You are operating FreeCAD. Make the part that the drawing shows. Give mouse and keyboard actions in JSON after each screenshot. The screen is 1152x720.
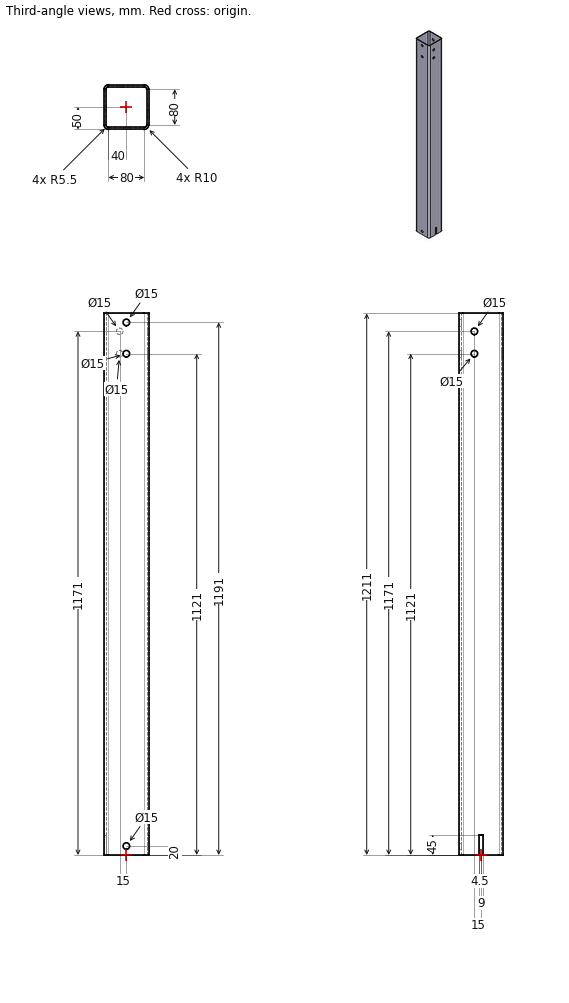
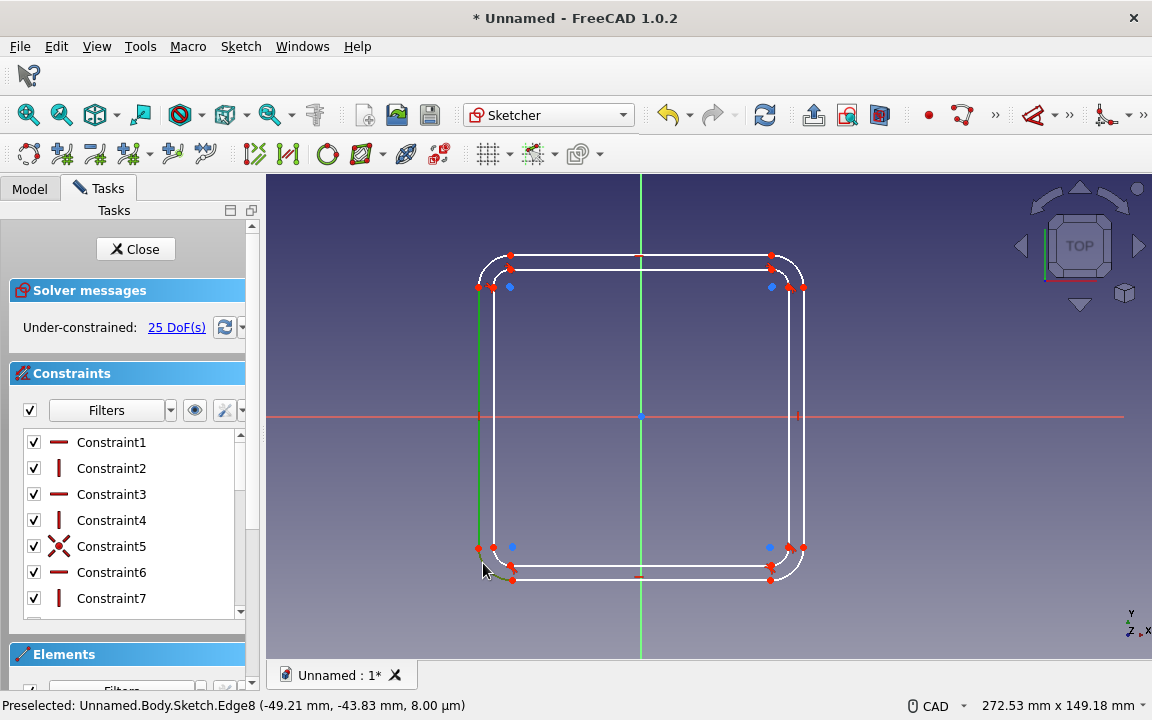
{"action": "key", "text": "t"}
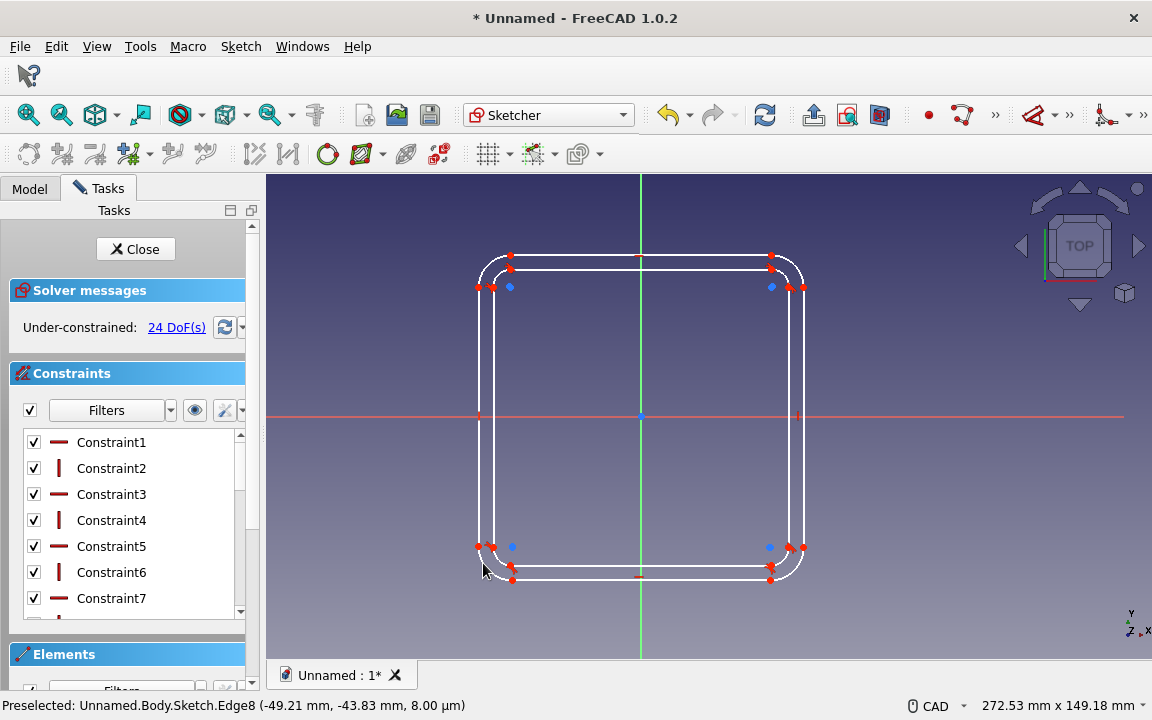
{"action": "left_click", "coordinate": [693, 566]}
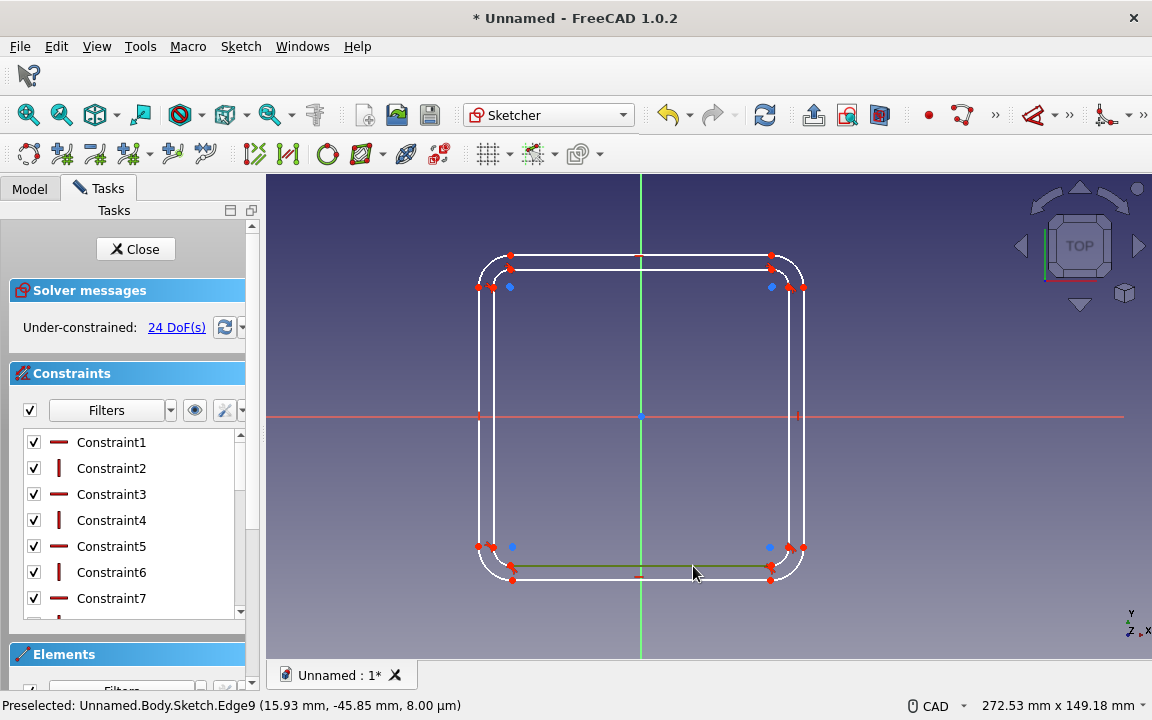
{"action": "left_click", "coordinate": [499, 560]}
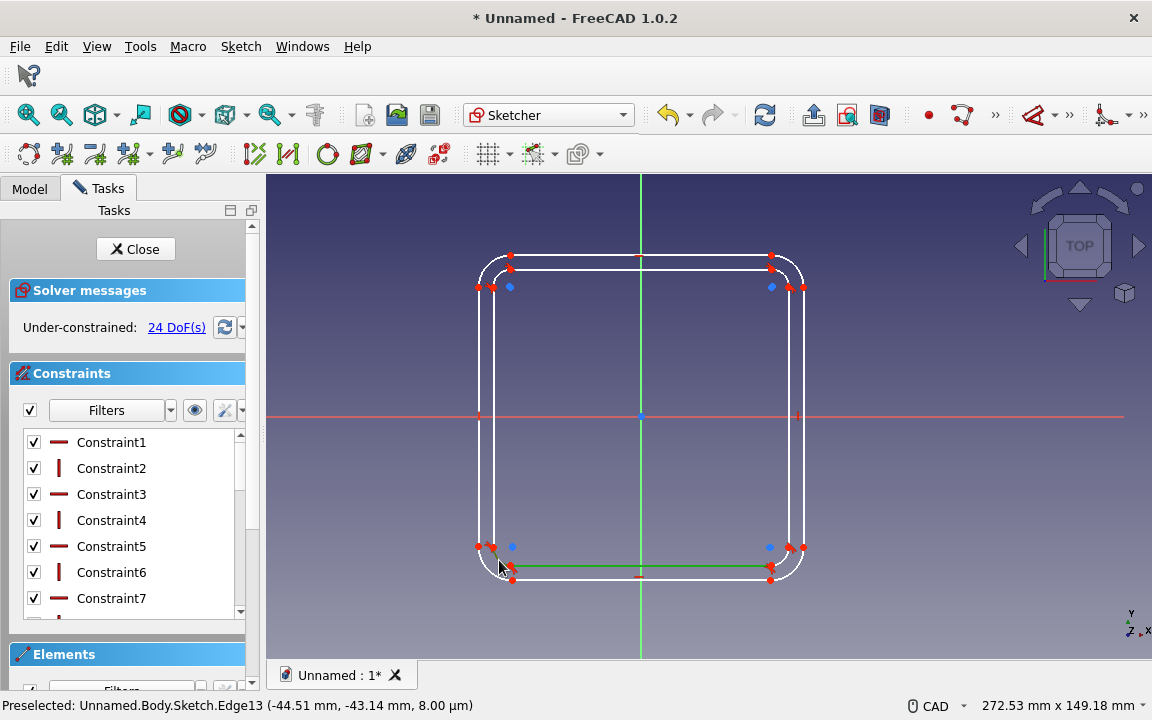
{"action": "key", "text": "t"}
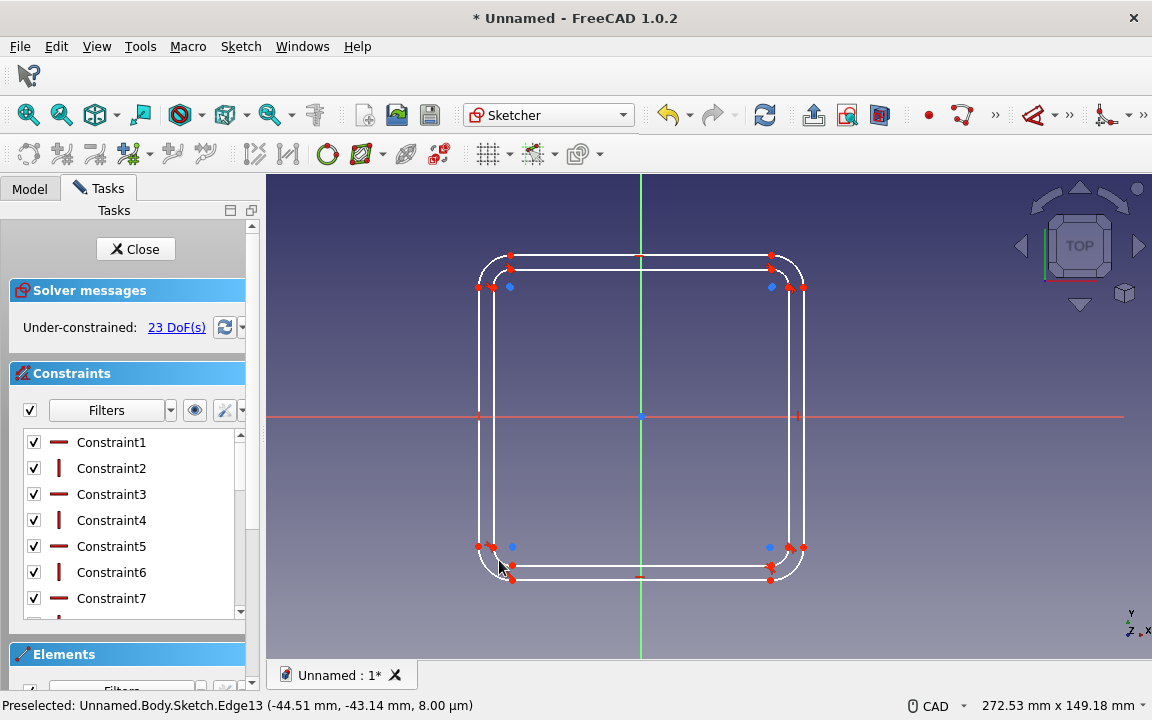
{"action": "left_click", "coordinate": [694, 566]}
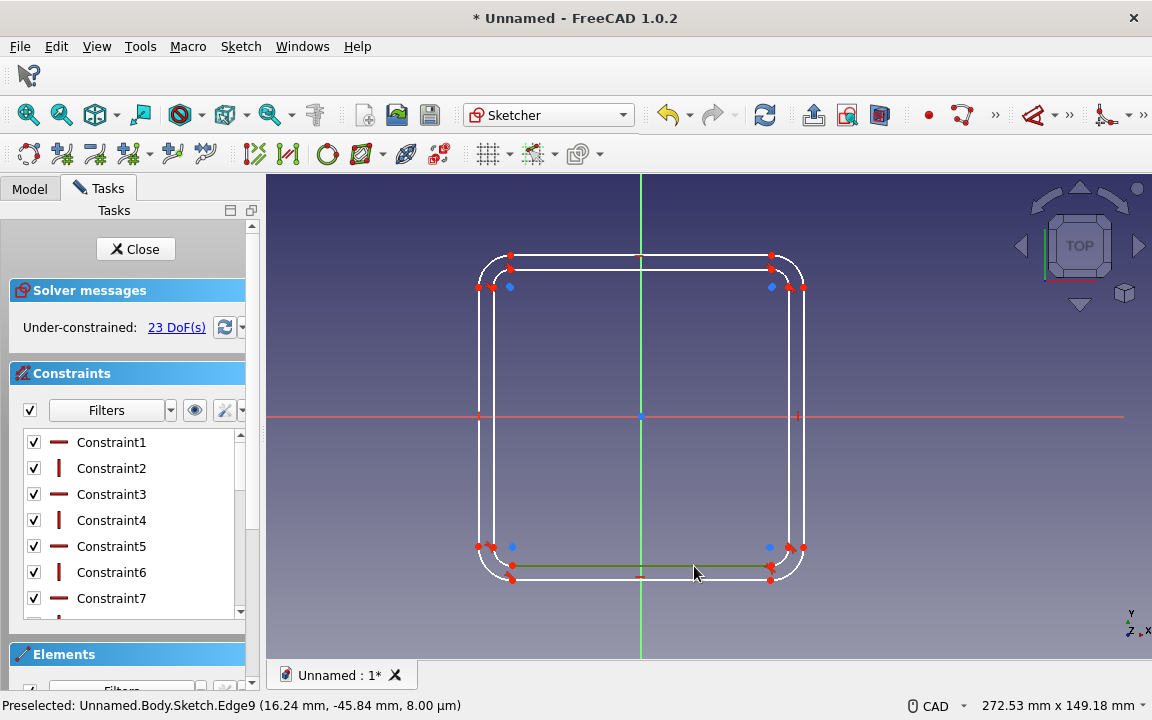
{"action": "left_click", "coordinate": [784, 560]}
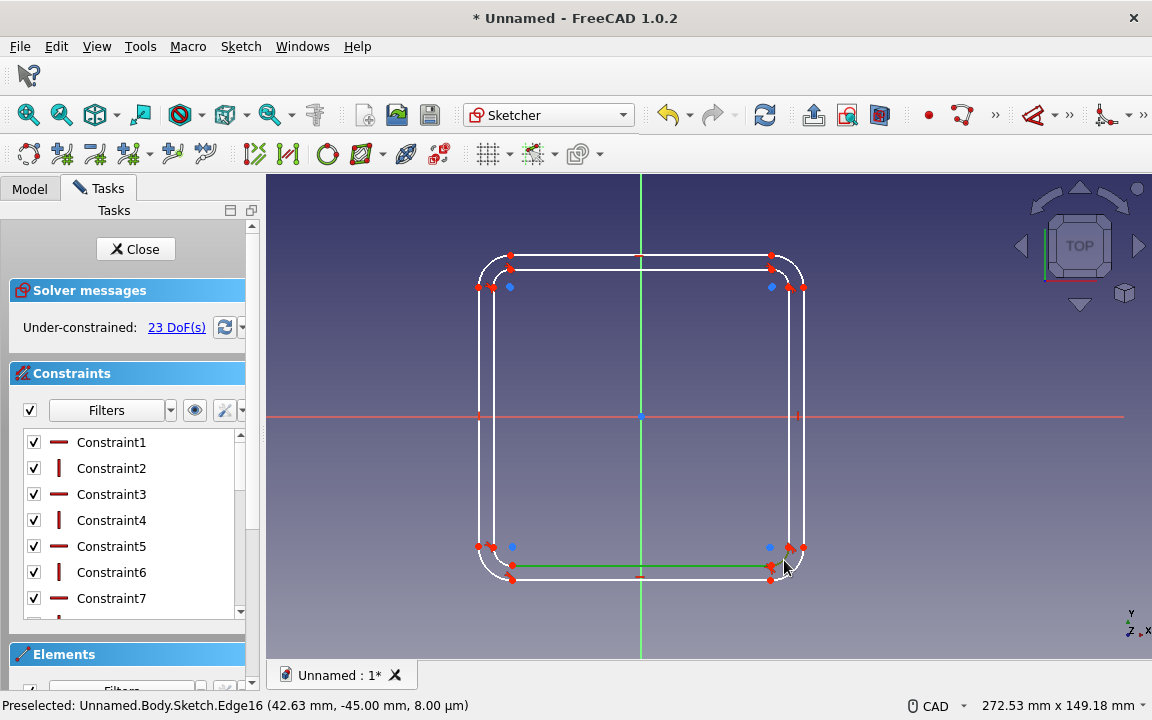
{"action": "key", "text": "t"}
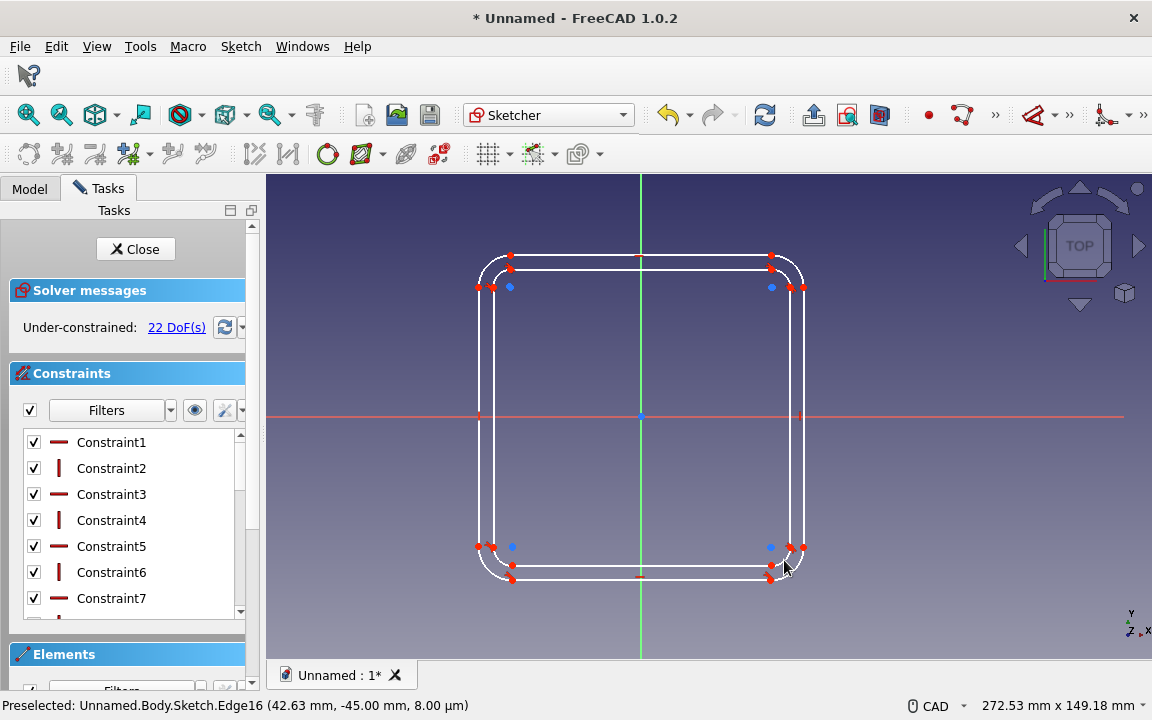
{"action": "left_click", "coordinate": [494, 470]}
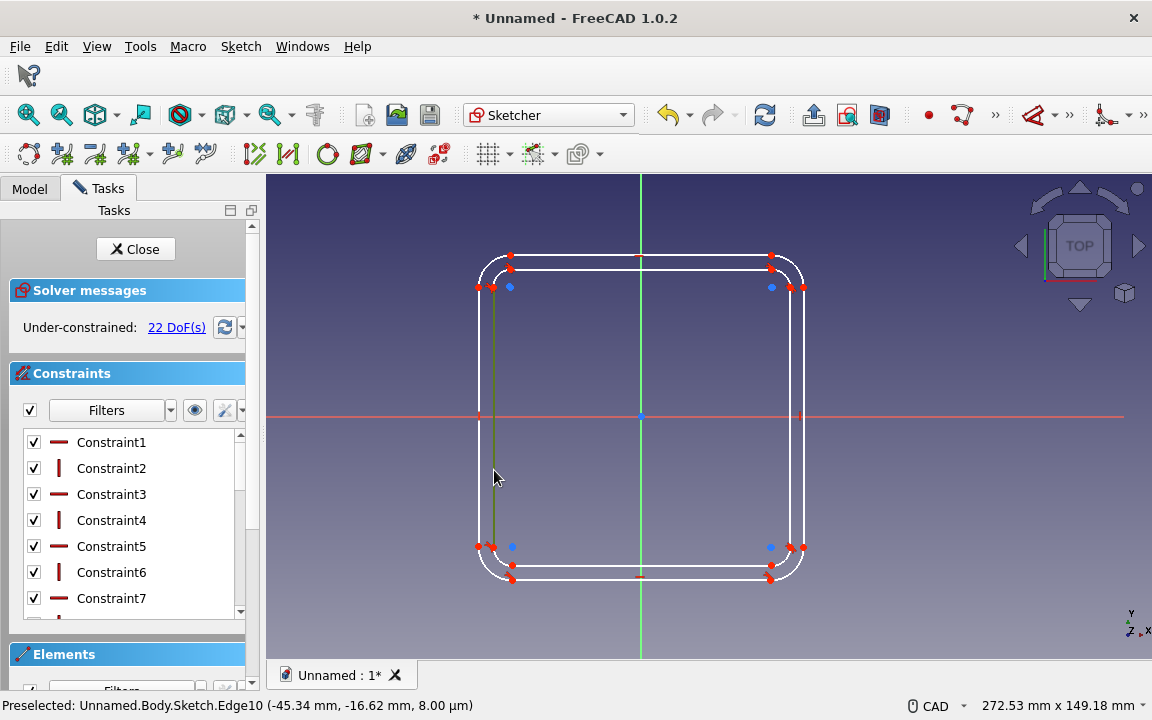
{"action": "left_click", "coordinate": [500, 561]}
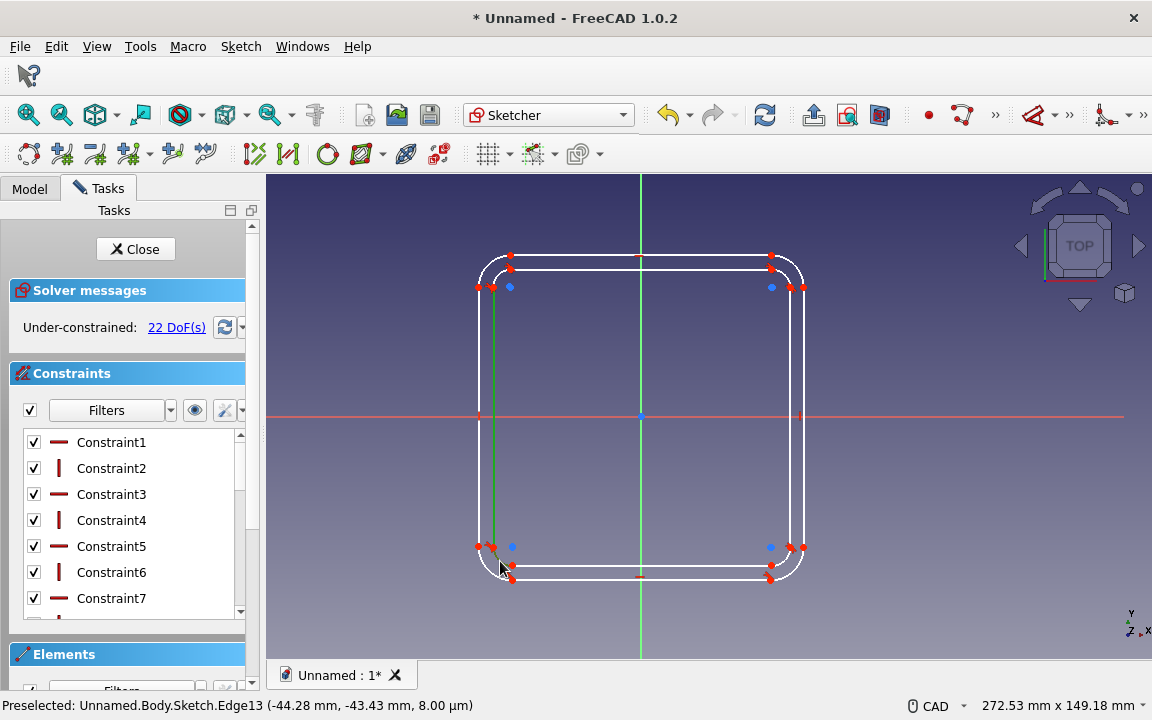
{"action": "key", "text": "t"}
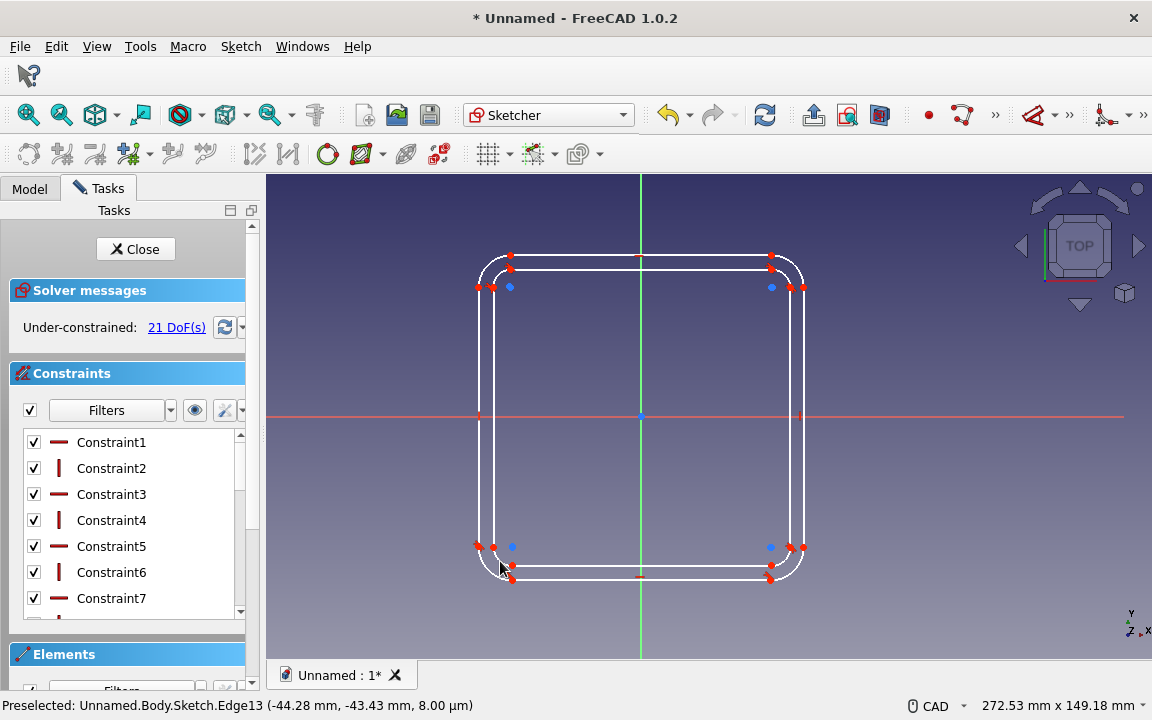
{"action": "left_click", "coordinate": [494, 470]}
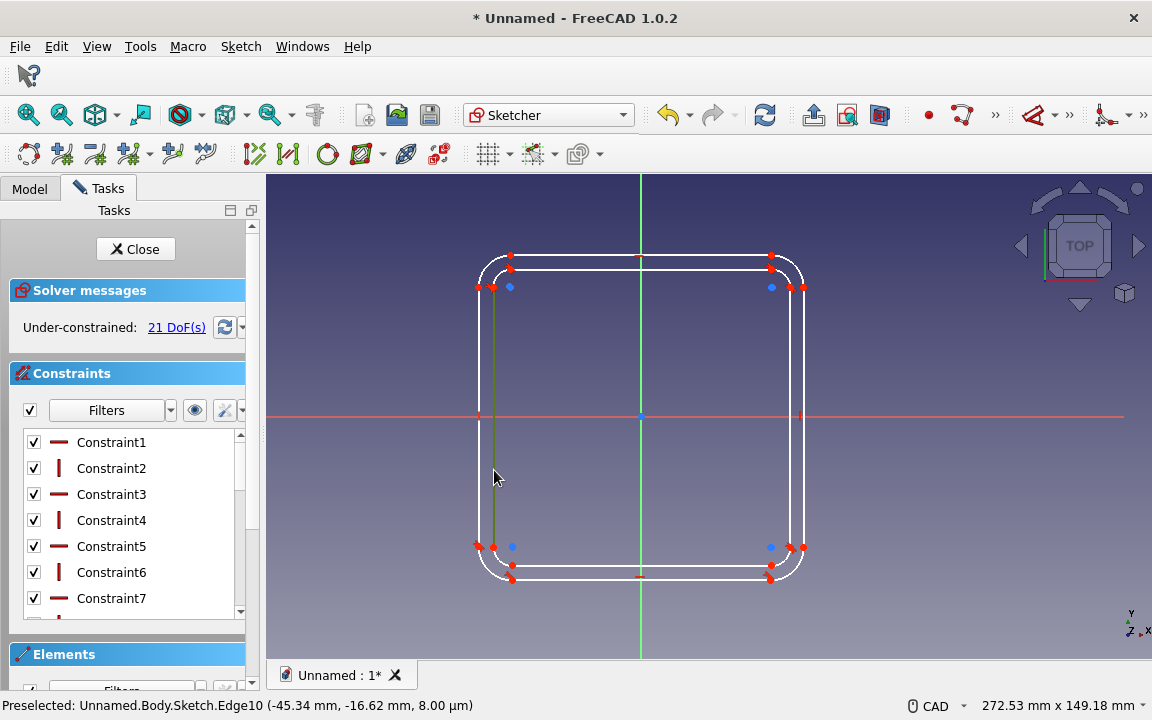
{"action": "left_click", "coordinate": [498, 275]}